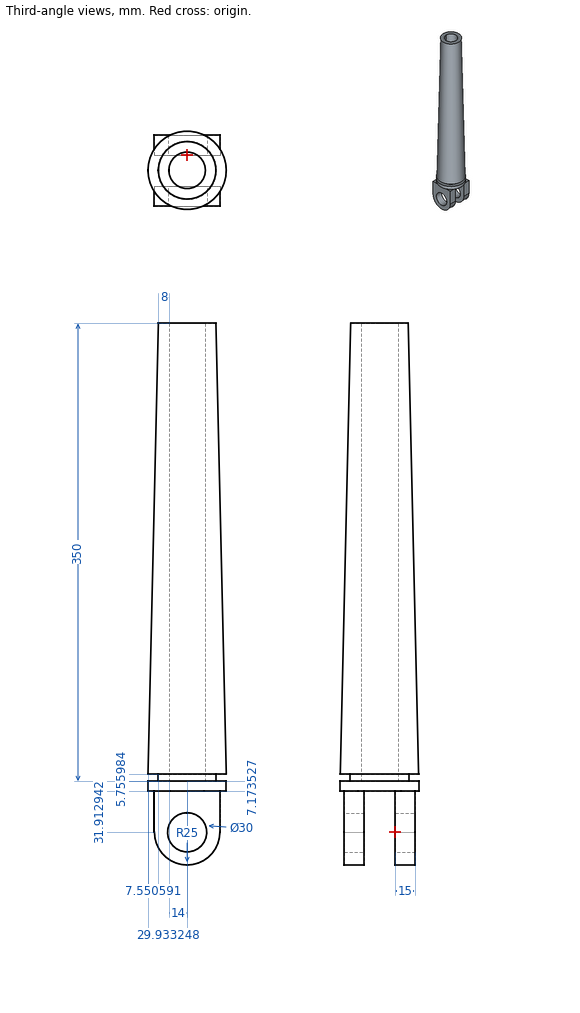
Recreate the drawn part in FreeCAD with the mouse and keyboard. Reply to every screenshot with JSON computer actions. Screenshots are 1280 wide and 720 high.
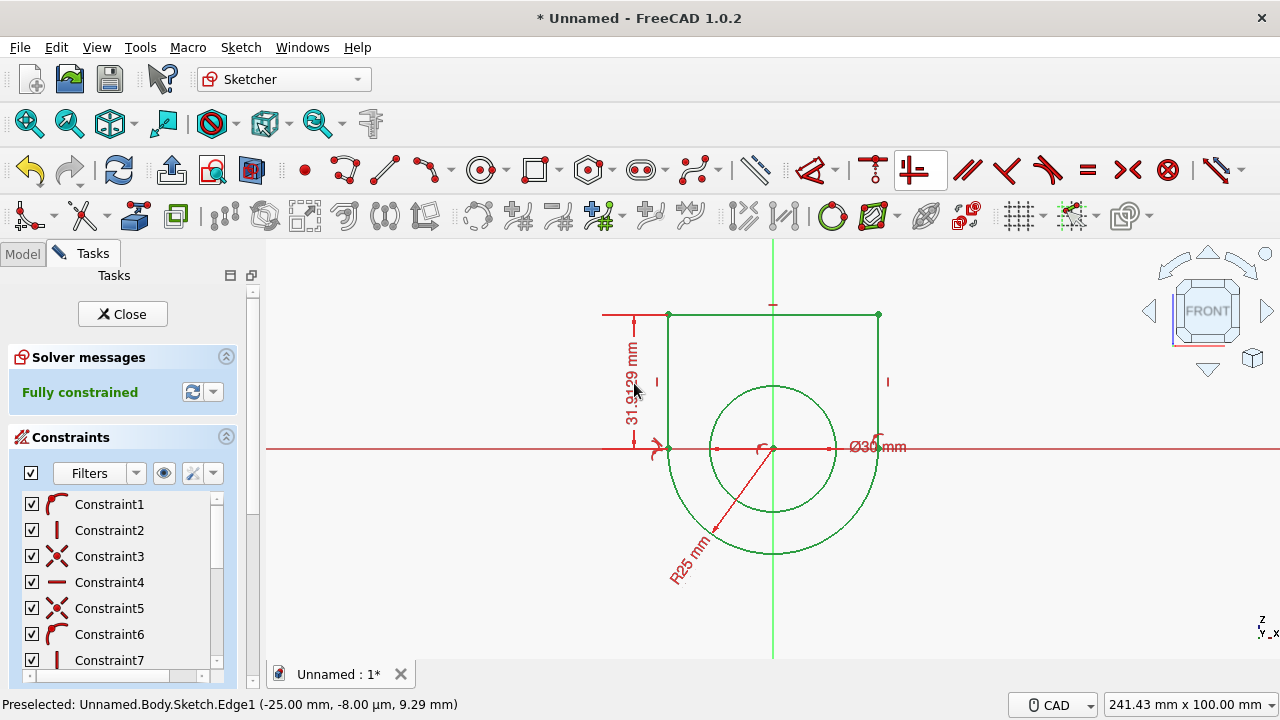
{"action": "left_click", "coordinate": [123, 314]}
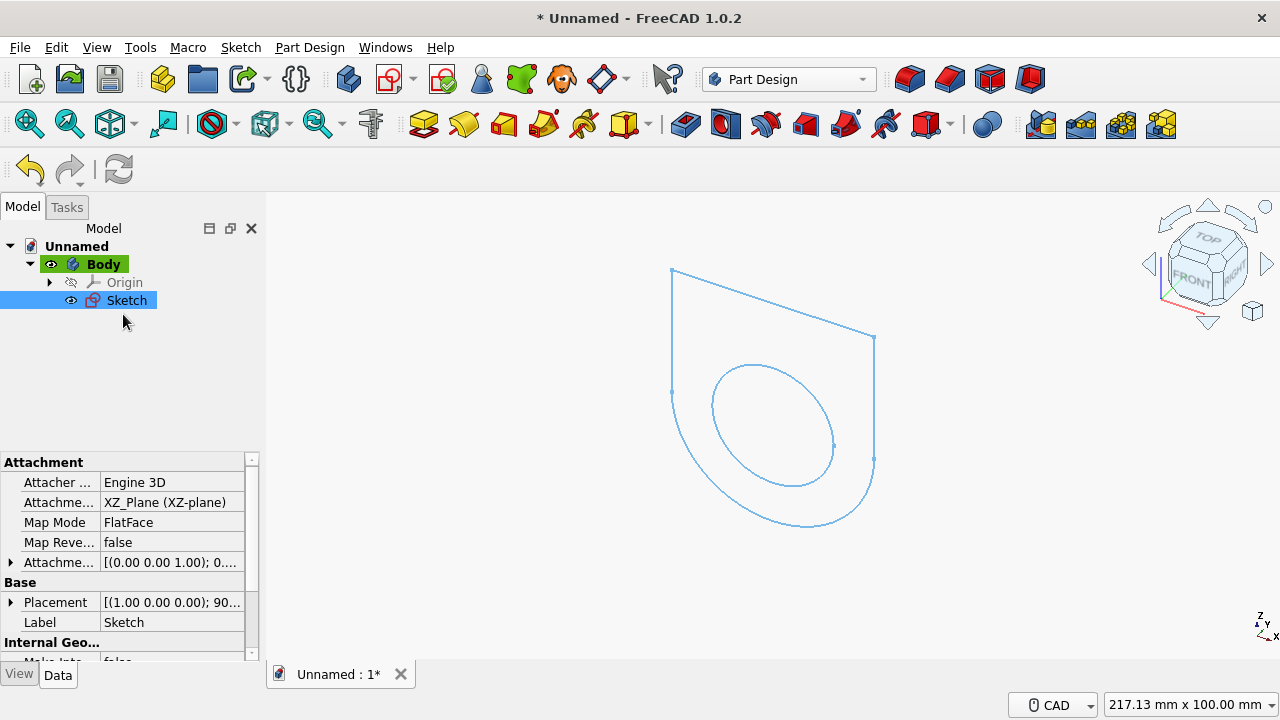
{"action": "left_click", "coordinate": [424, 124]}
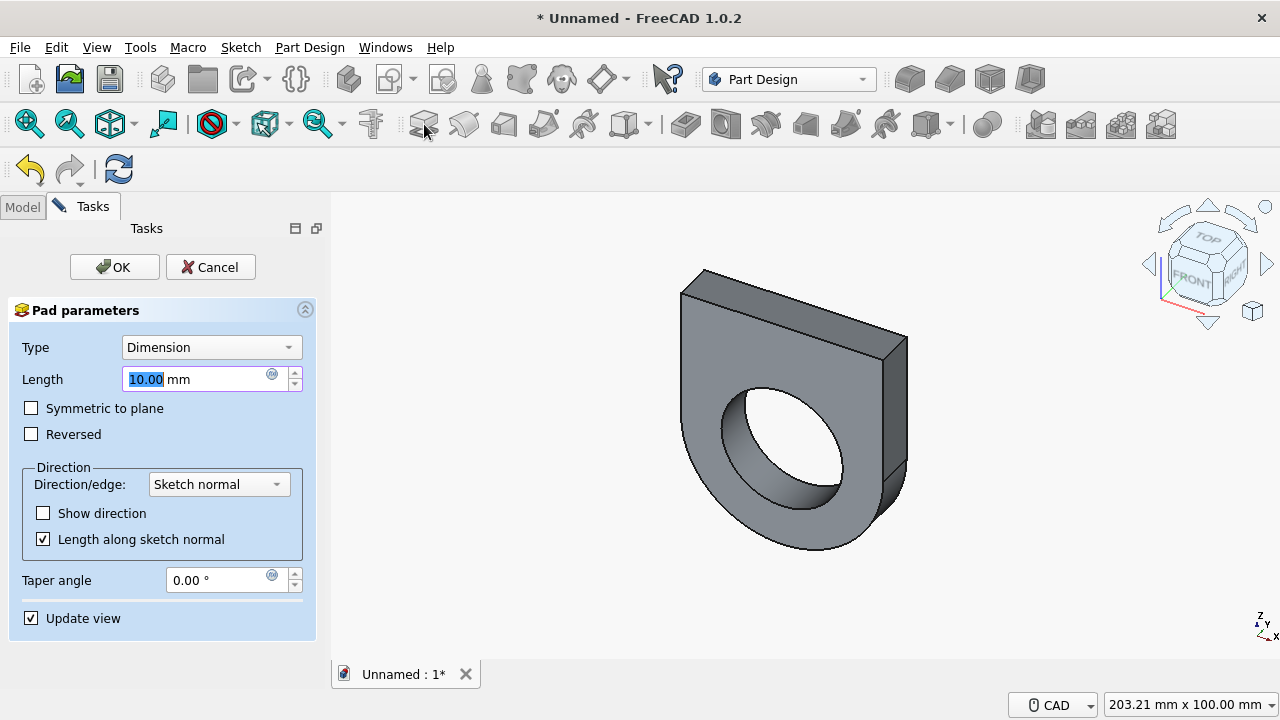
{"action": "type", "text": "15"}
{"action": "key", "text": "Tab"}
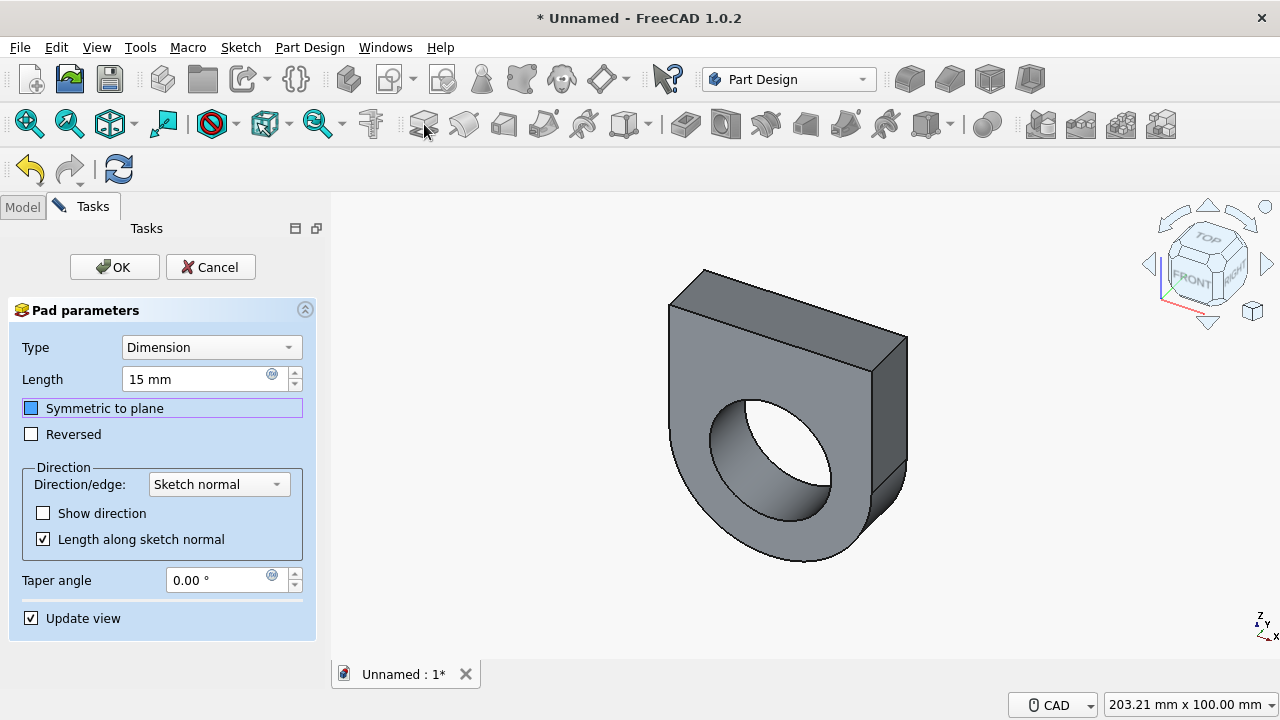
{"action": "left_click", "coordinate": [30, 434]}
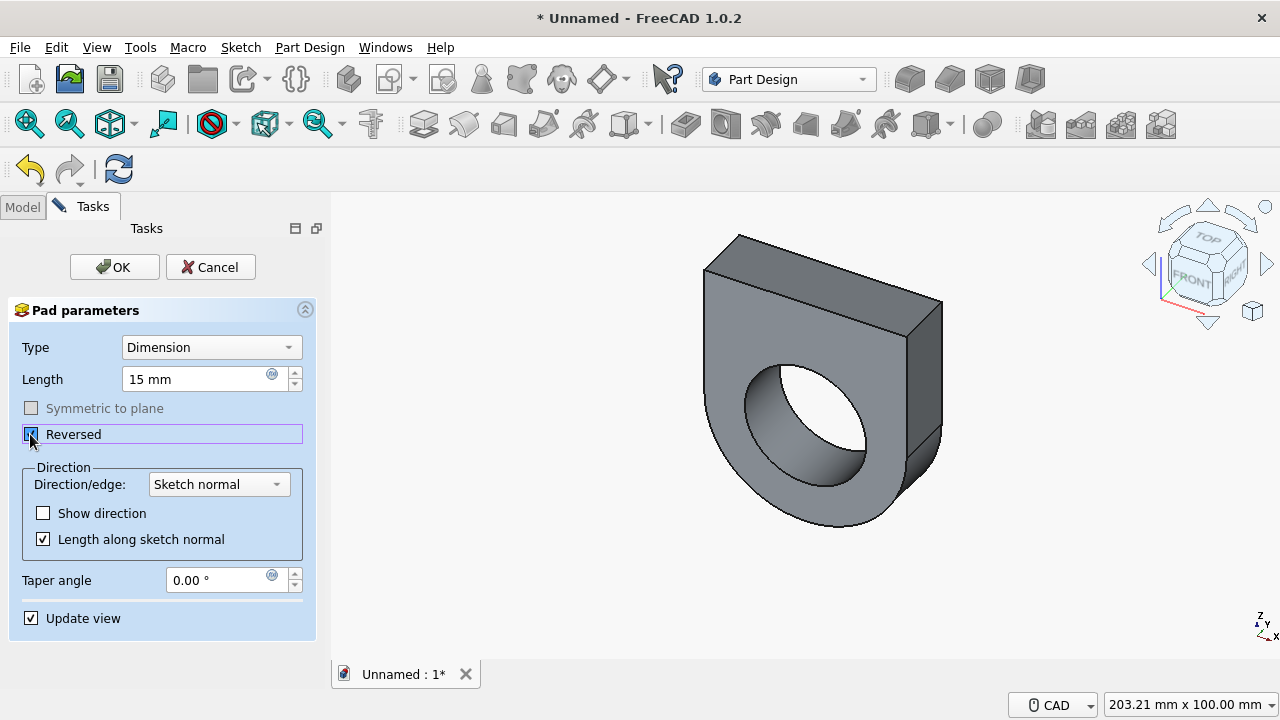
{"action": "left_click", "coordinate": [115, 267]}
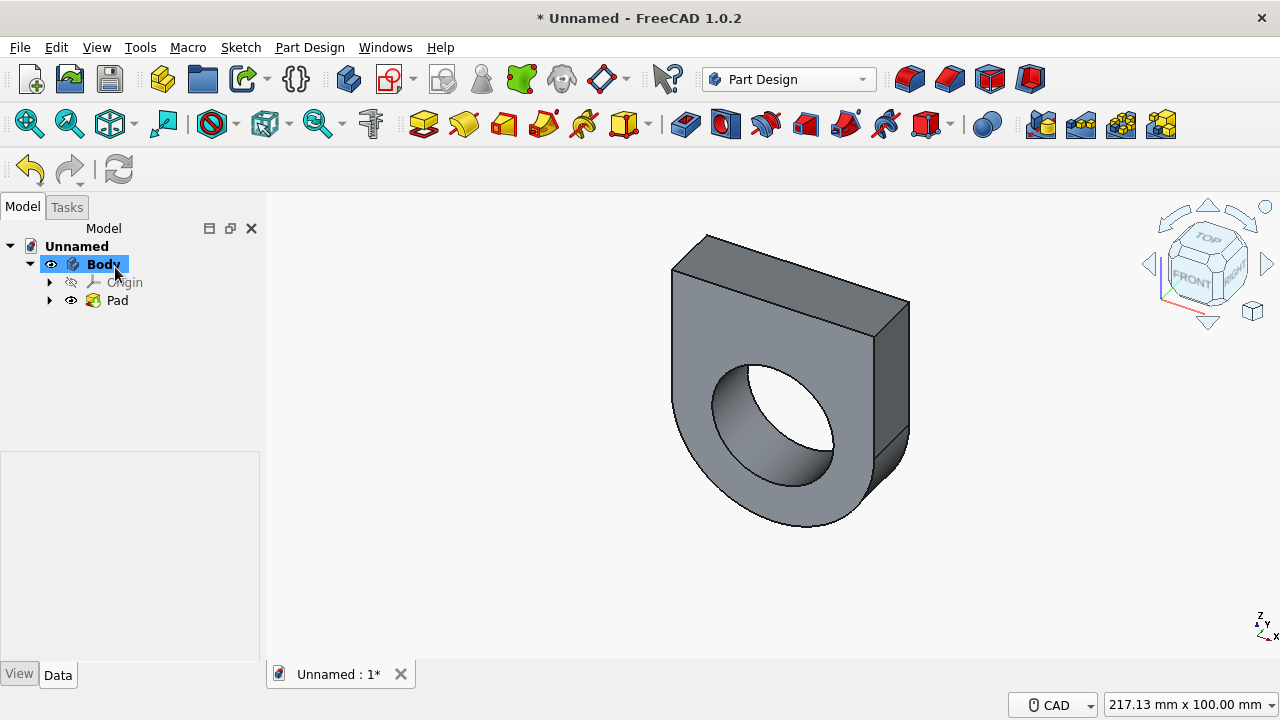
{"action": "left_click", "coordinate": [50, 282]}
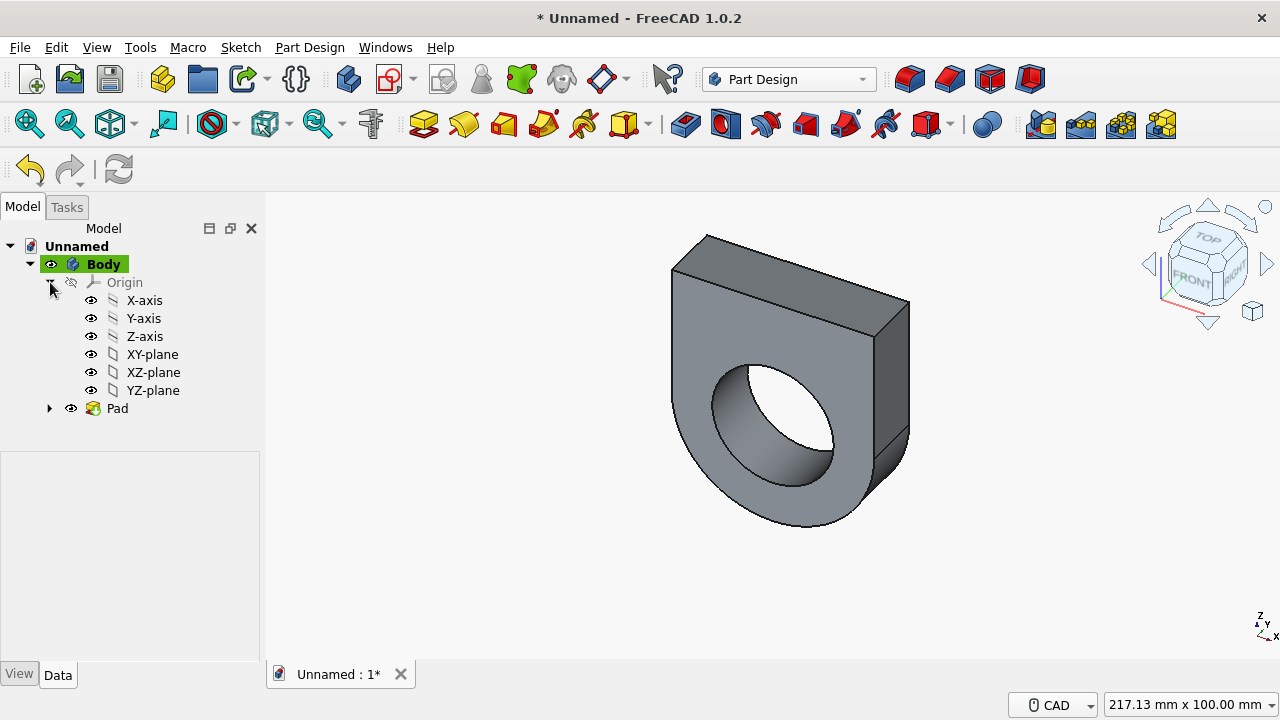
{"action": "left_click", "coordinate": [136, 372]}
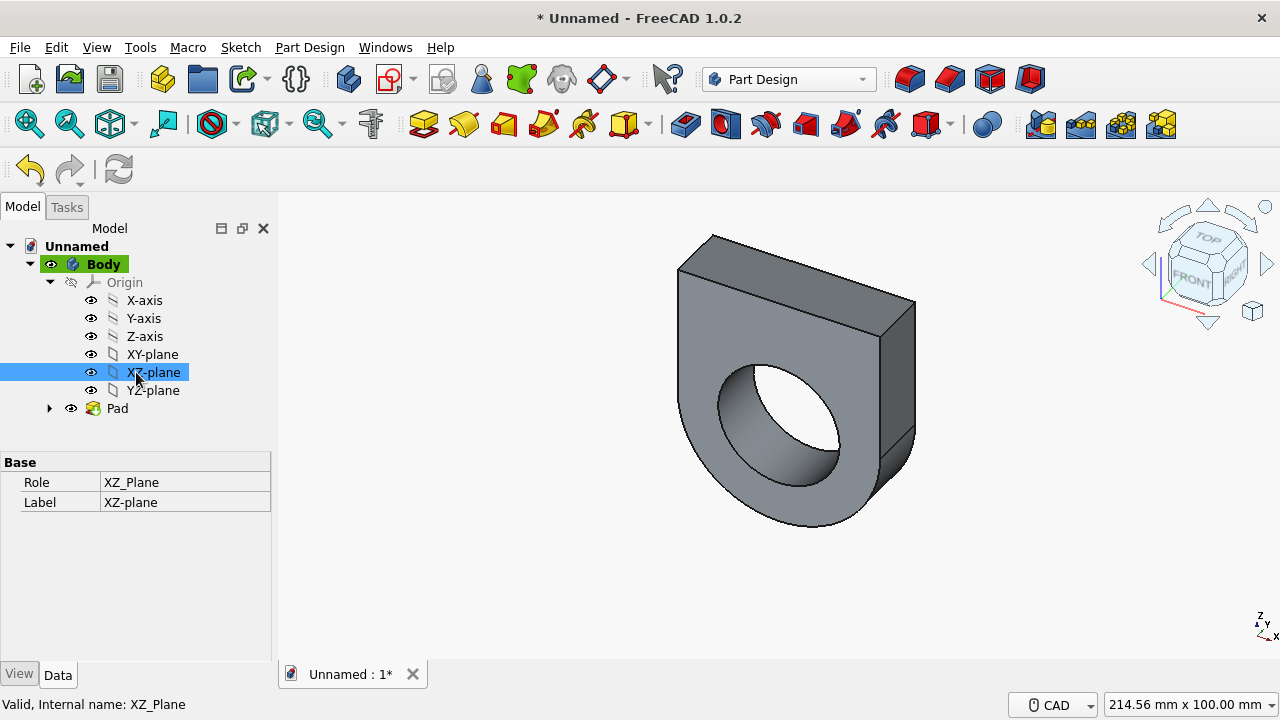
{"action": "left_click", "coordinate": [602, 80]}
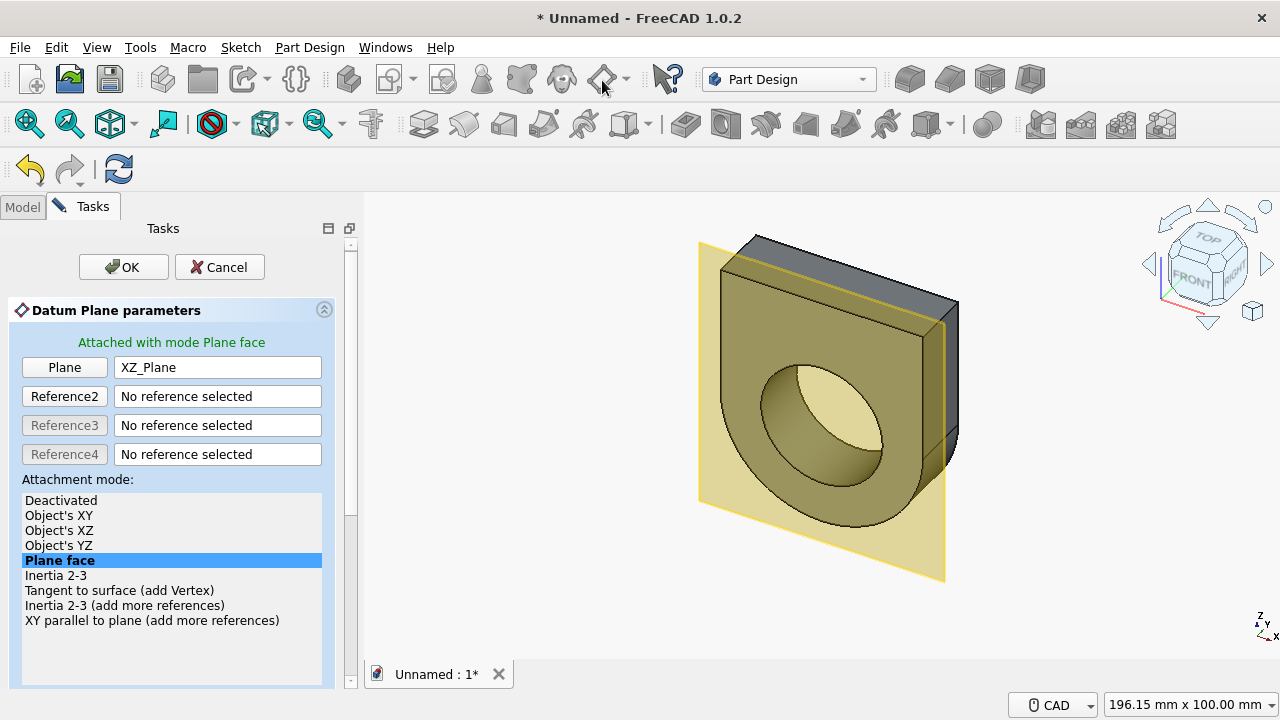
{"action": "scroll", "coordinate": [351, 463], "scroll_direction": "down", "scroll_amount": 3}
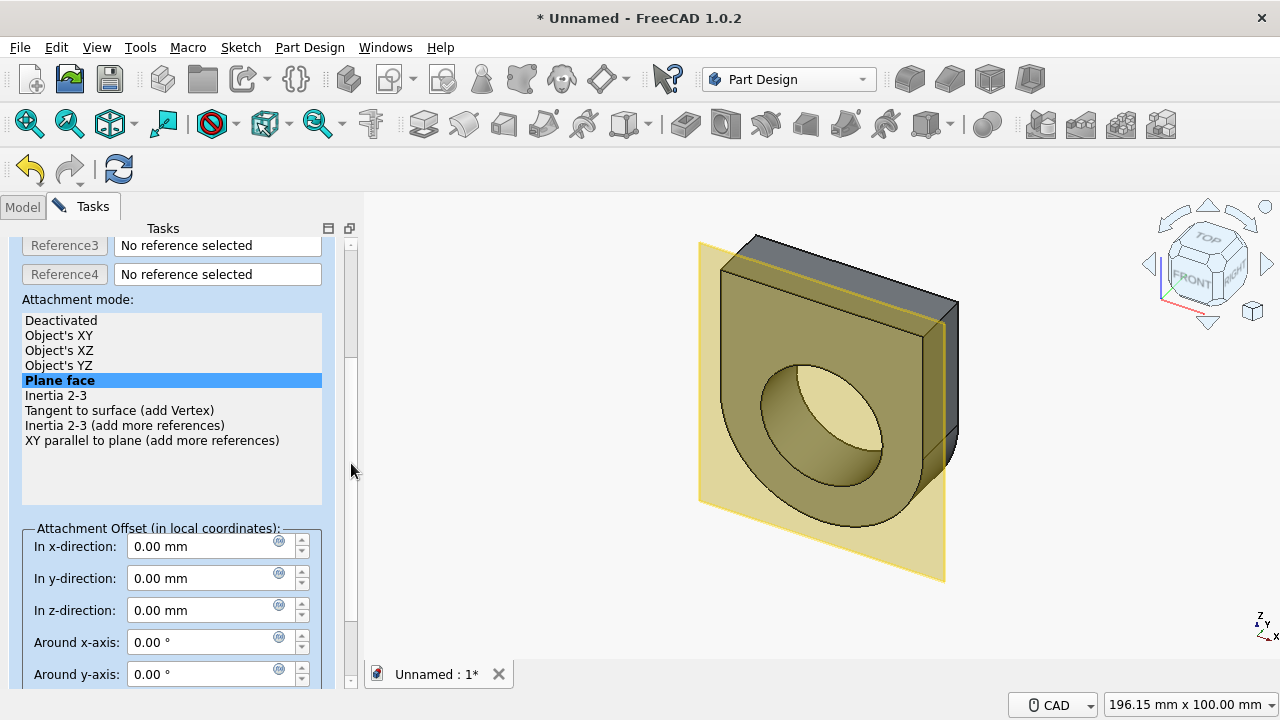
{"action": "triple_click", "coordinate": [210, 610]}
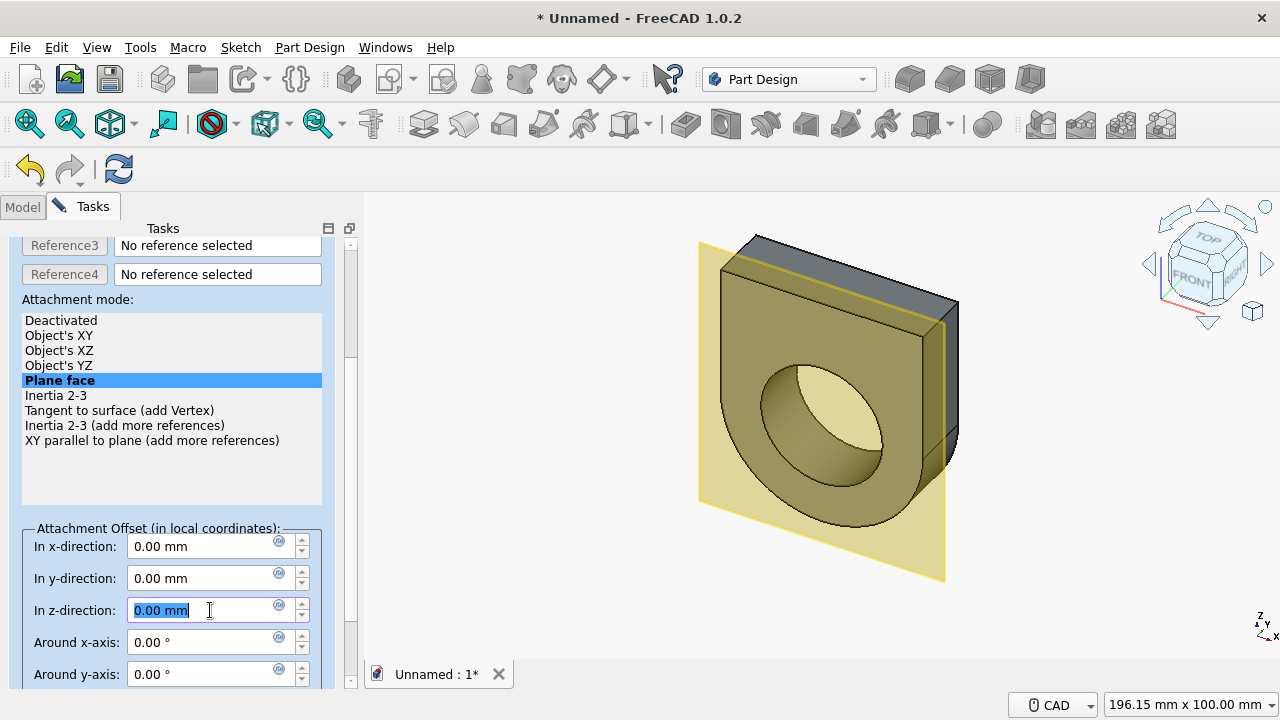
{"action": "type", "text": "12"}
{"action": "key", "text": "Tab"}